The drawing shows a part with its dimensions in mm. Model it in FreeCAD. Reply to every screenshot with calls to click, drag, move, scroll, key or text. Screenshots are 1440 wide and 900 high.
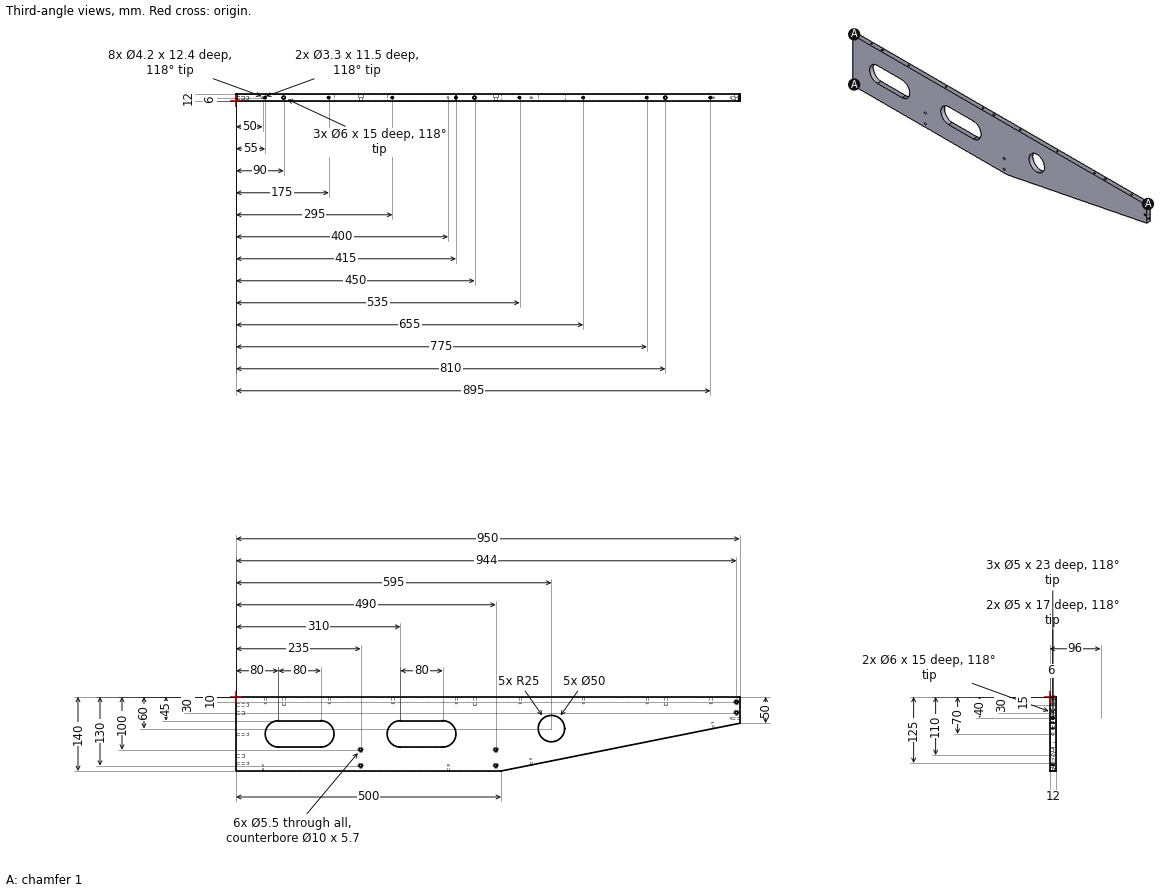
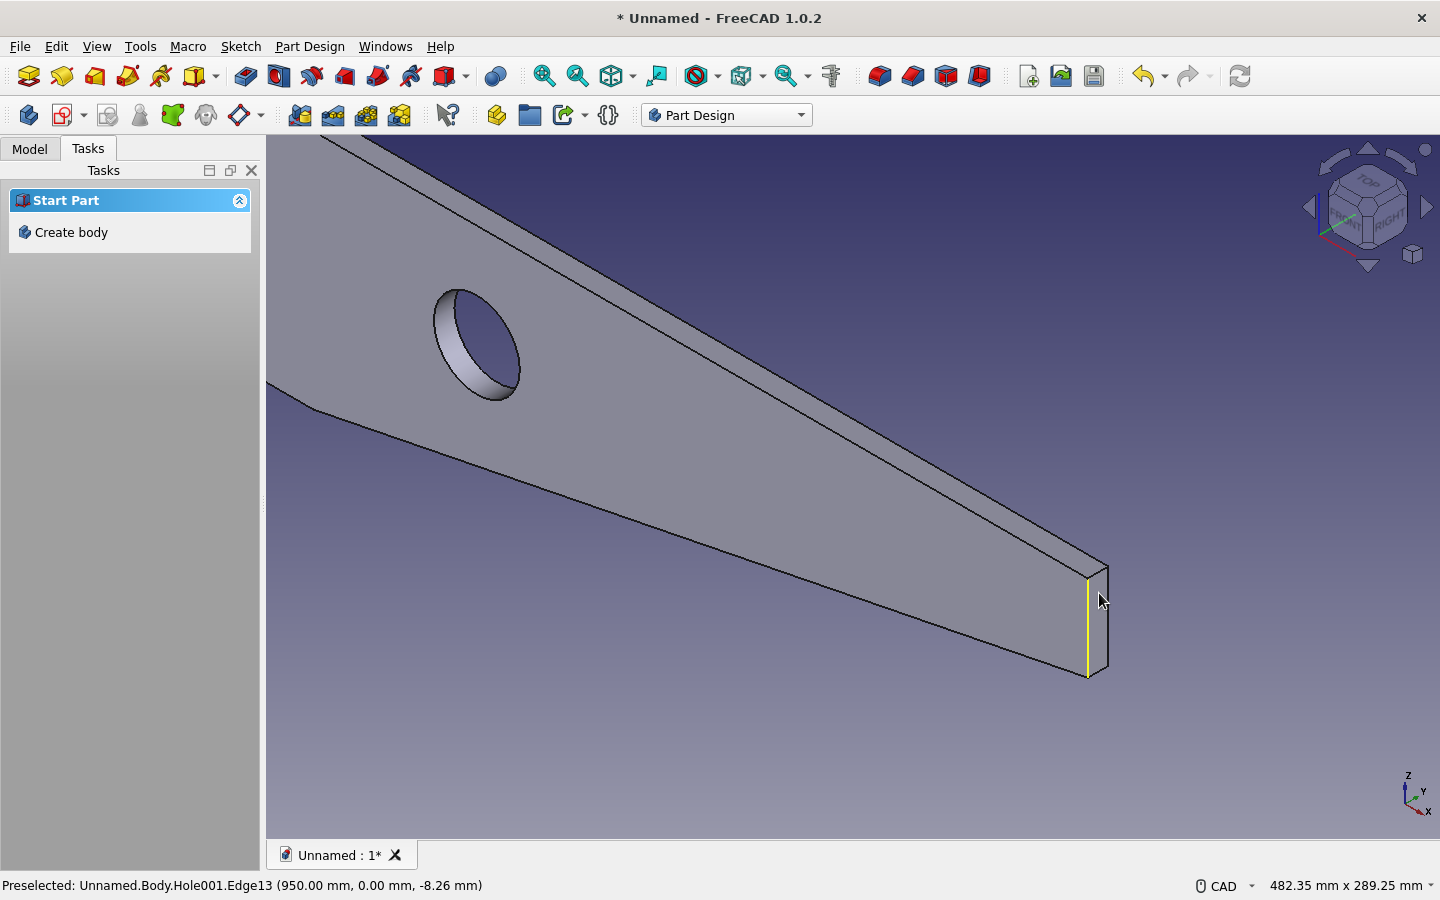
click(1098, 593)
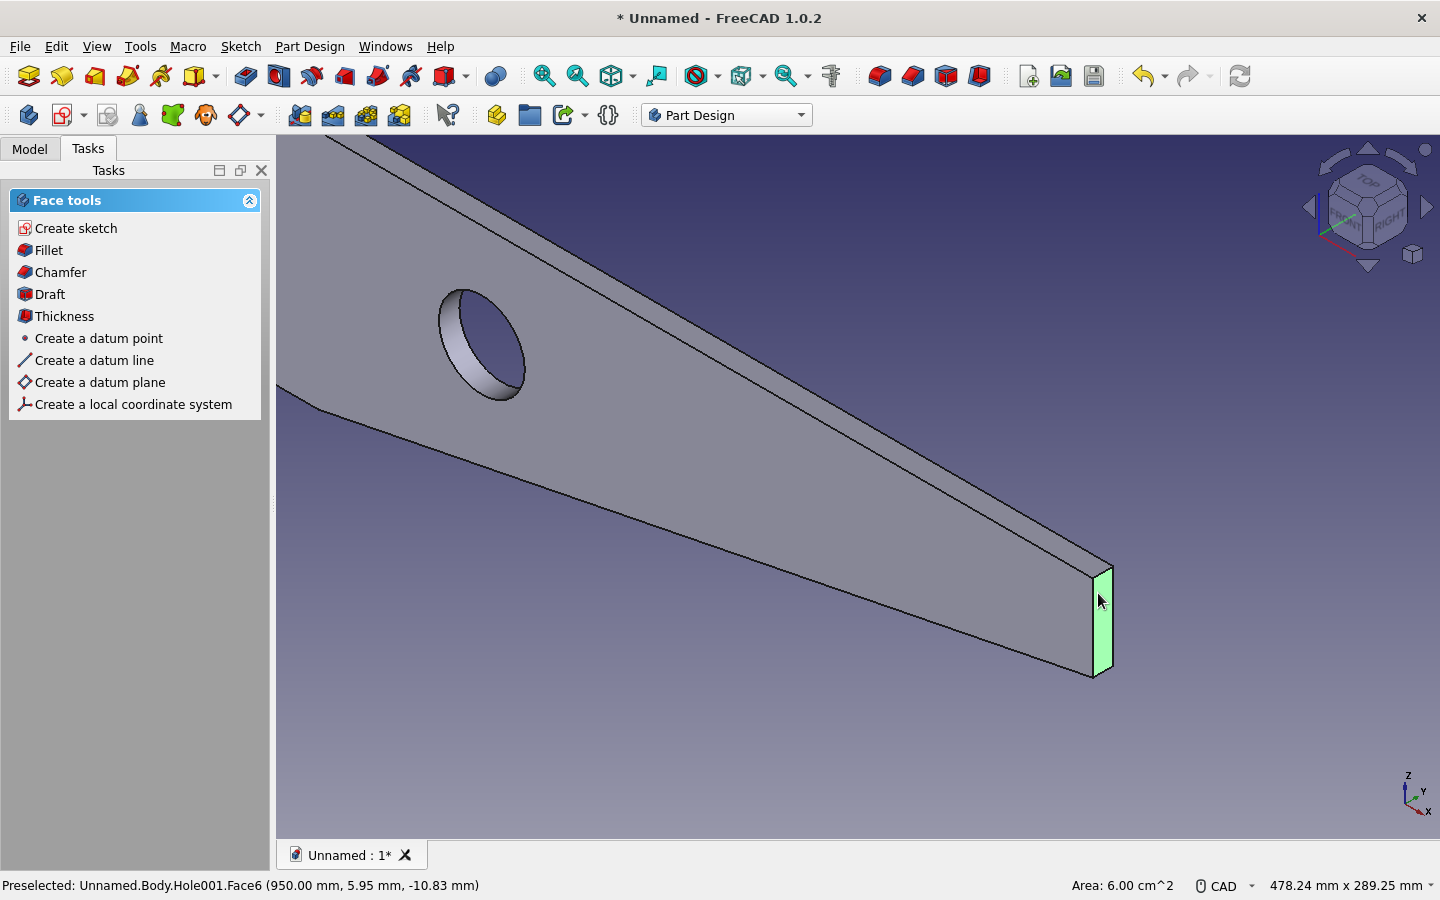
click(62, 116)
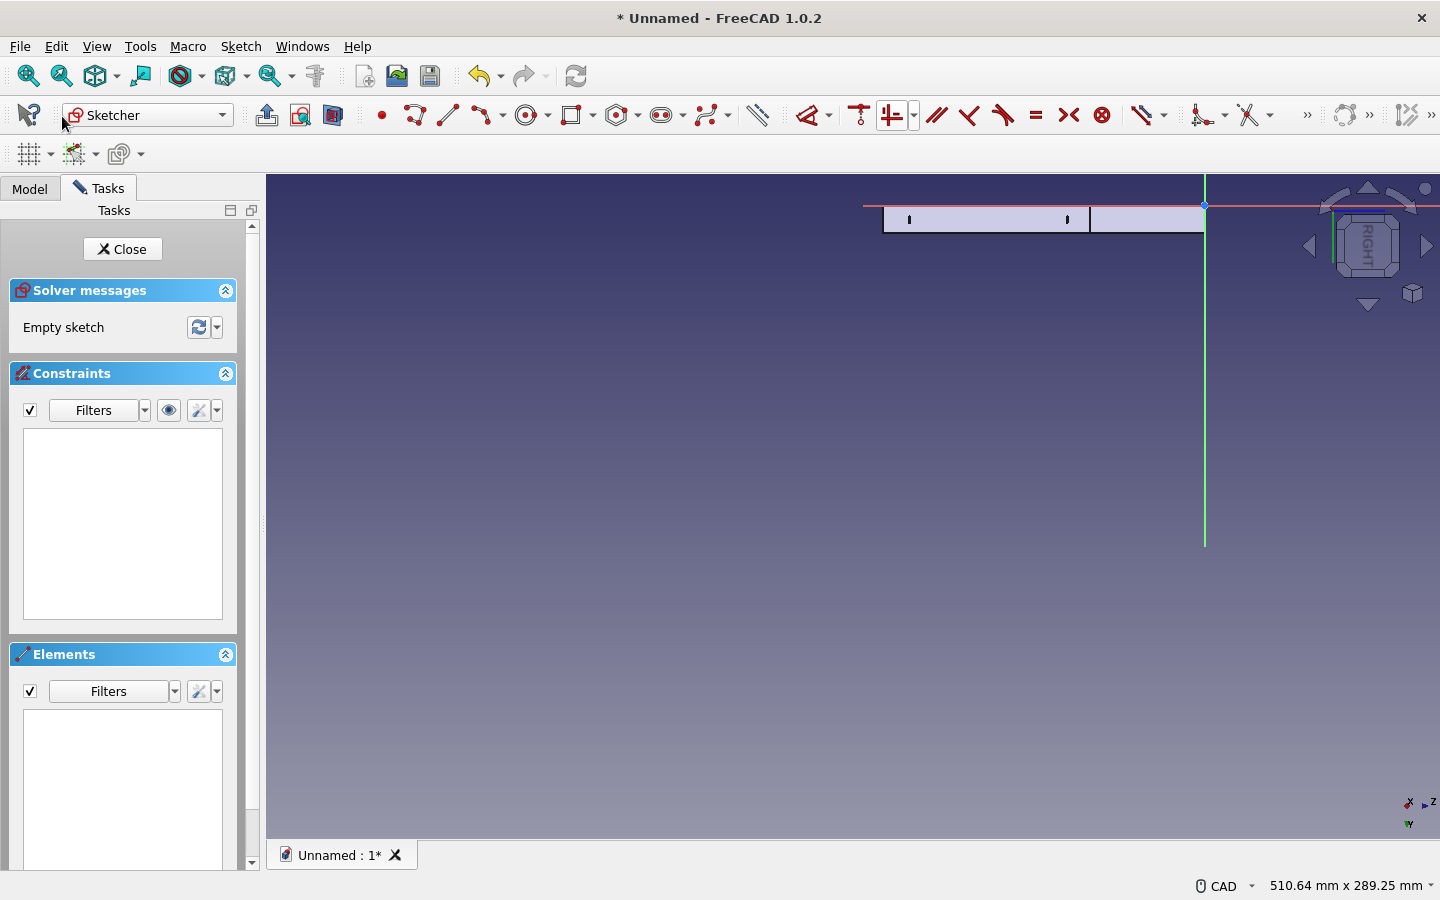
scroll(784, 506, down, 5)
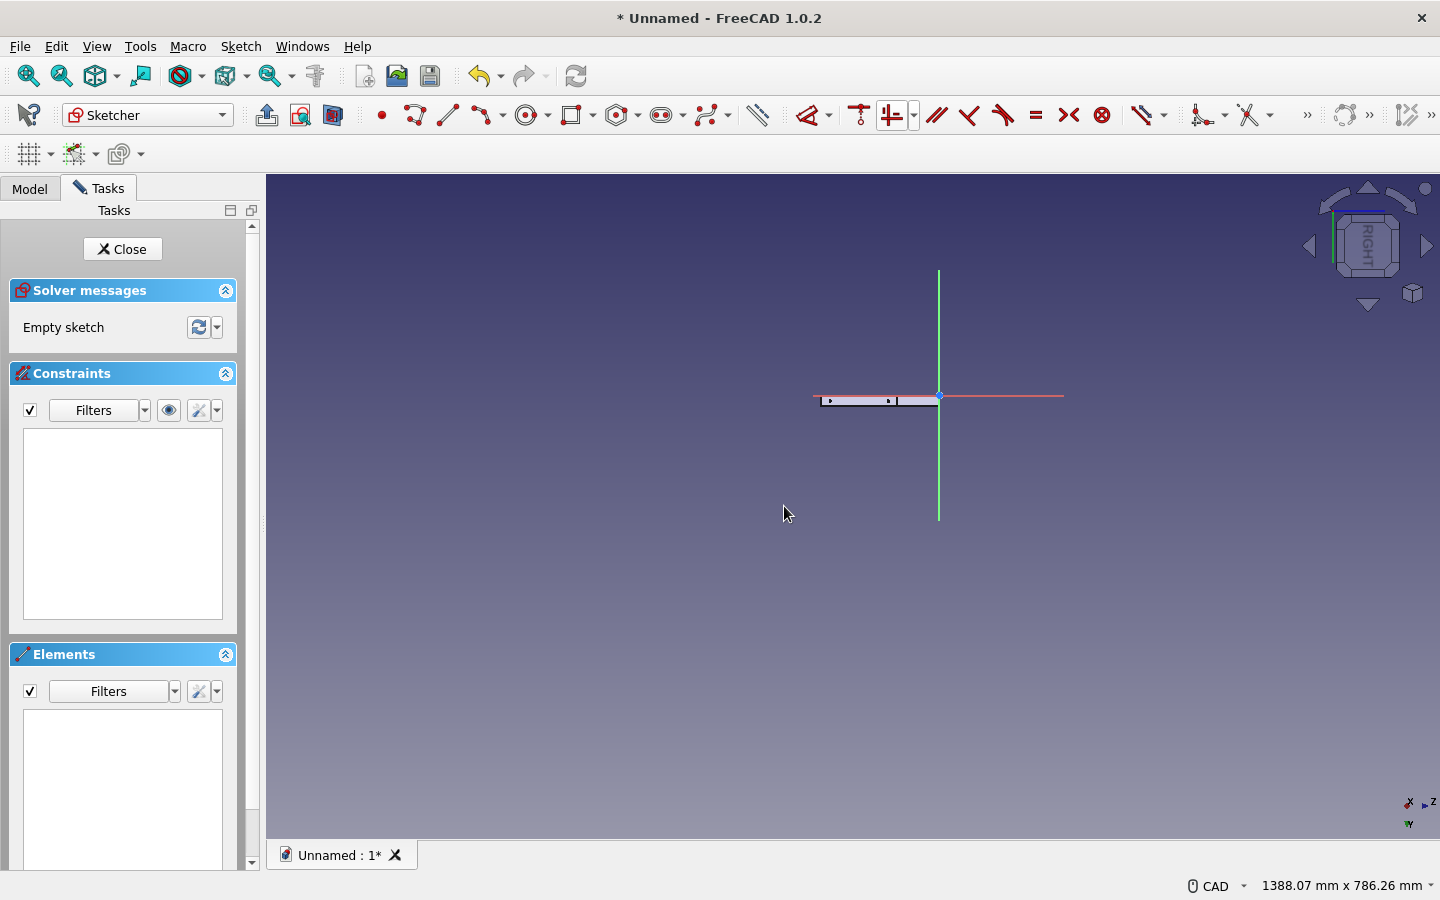
scroll(956, 420, up, 8)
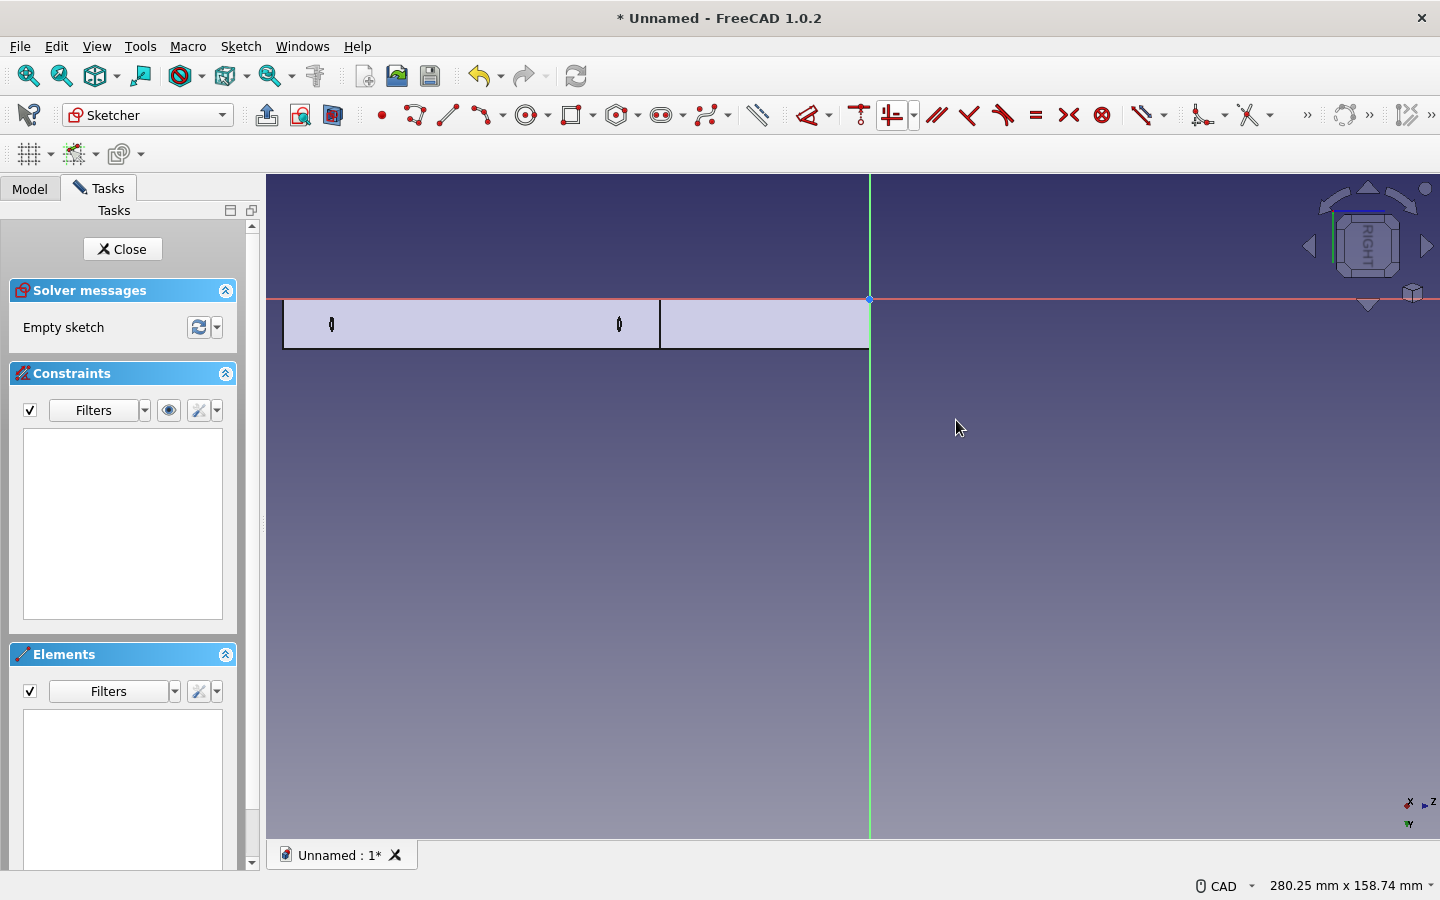
click(526, 116)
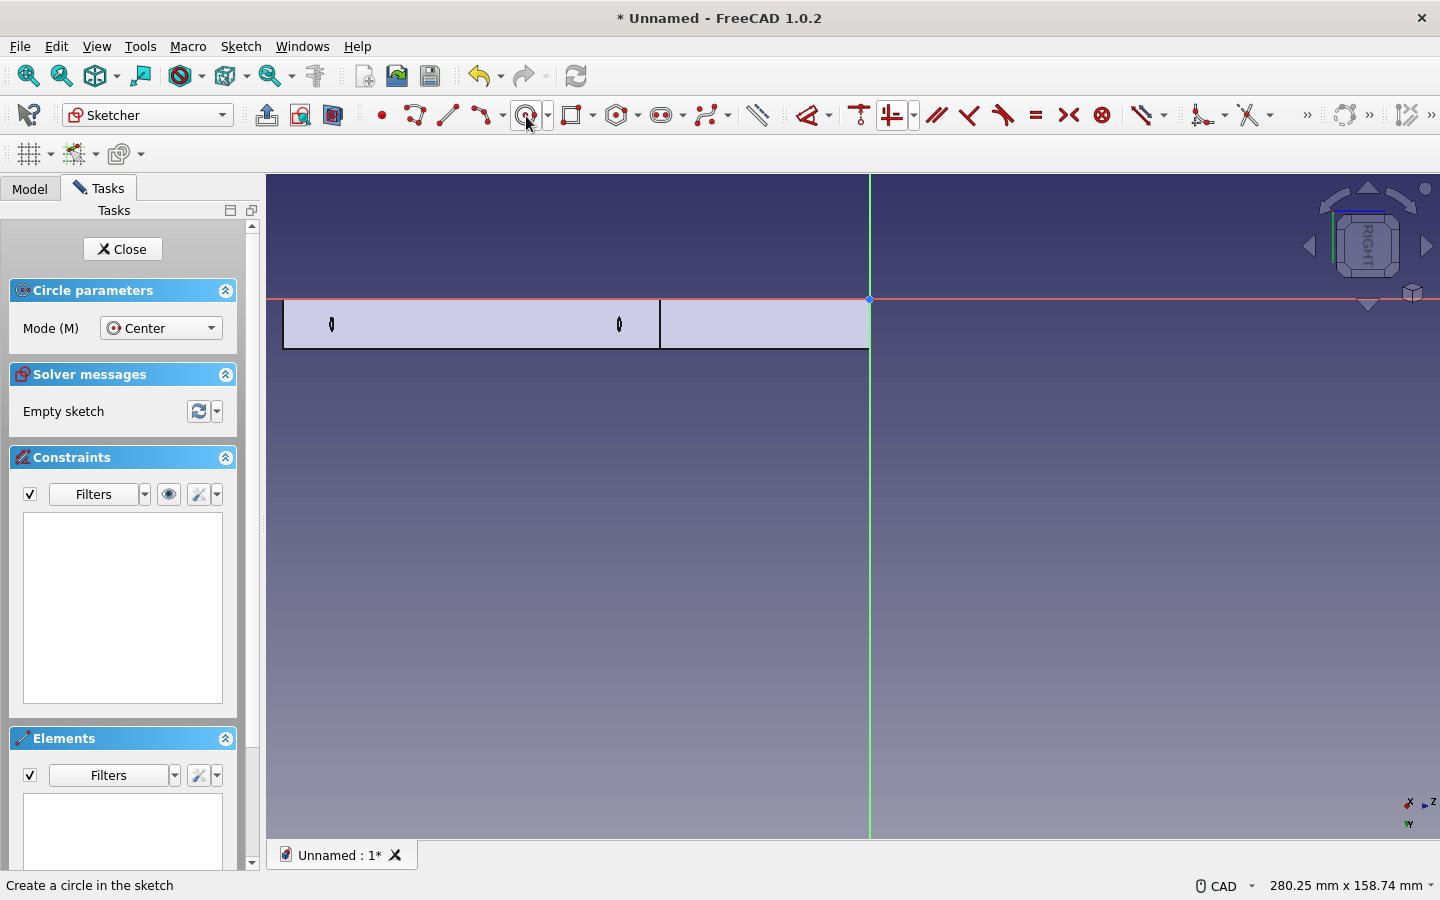
scroll(702, 324, up, 4)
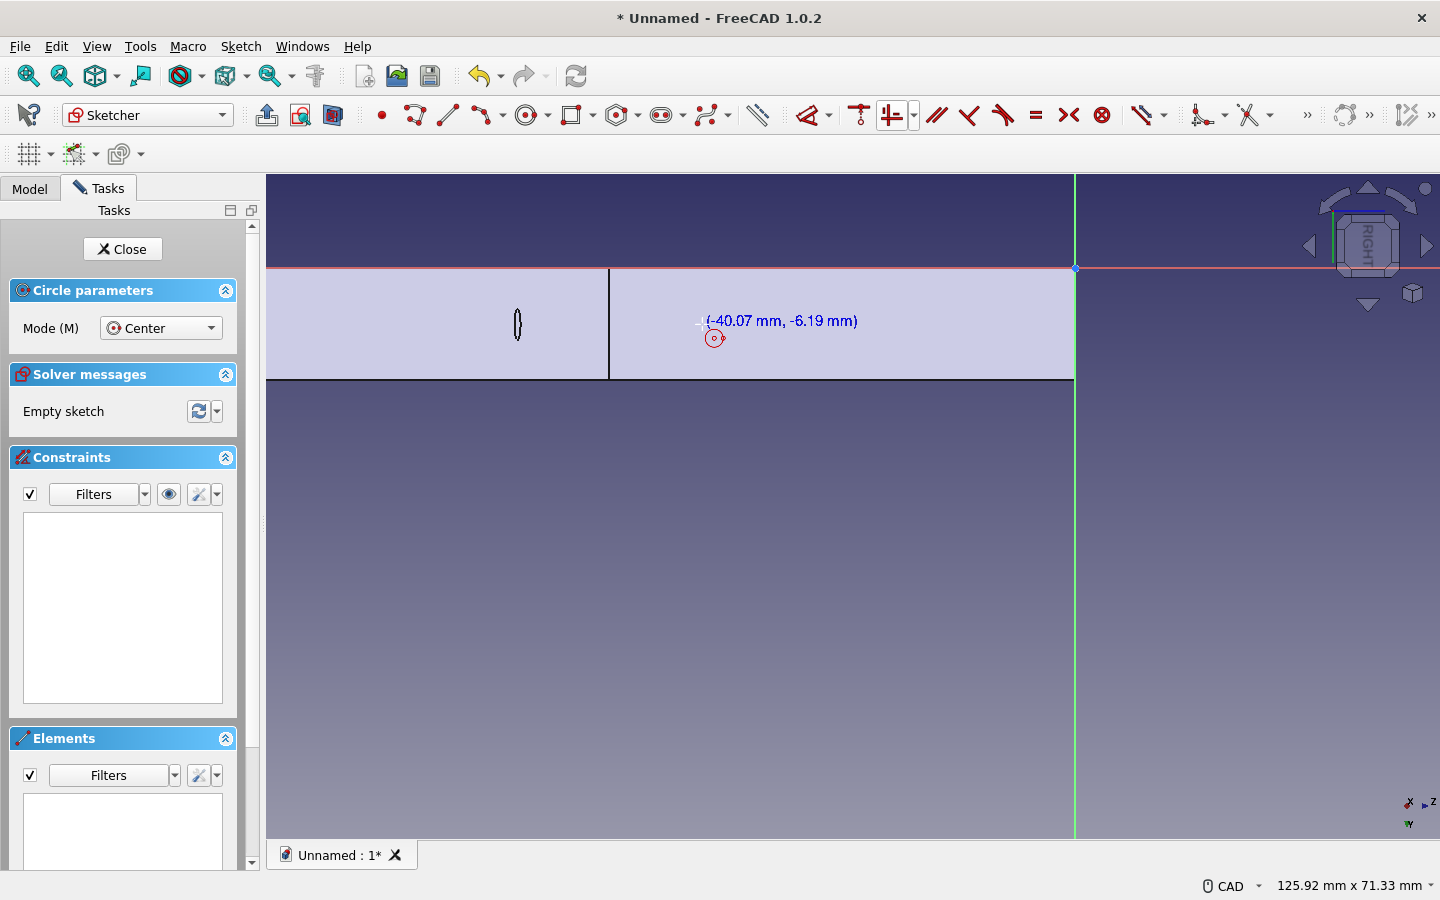
click(702, 324)
move(719, 308)